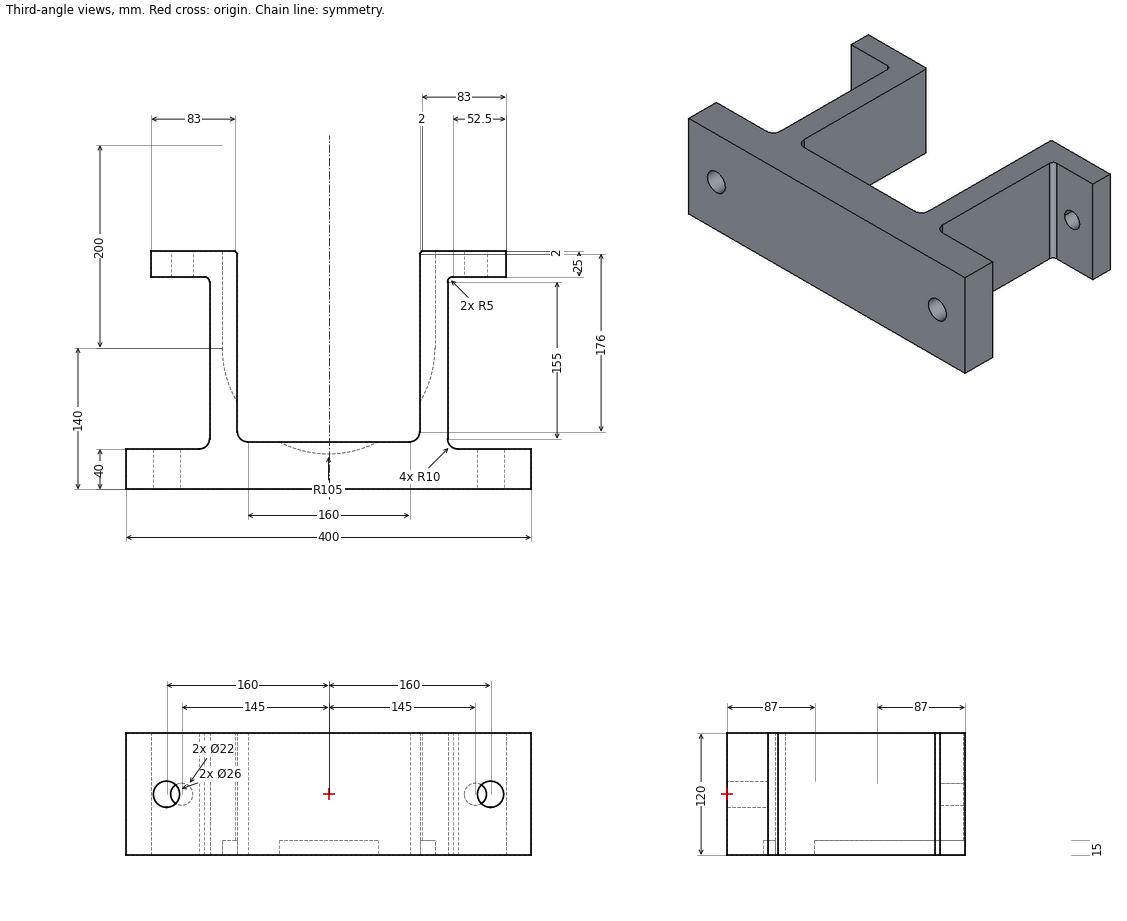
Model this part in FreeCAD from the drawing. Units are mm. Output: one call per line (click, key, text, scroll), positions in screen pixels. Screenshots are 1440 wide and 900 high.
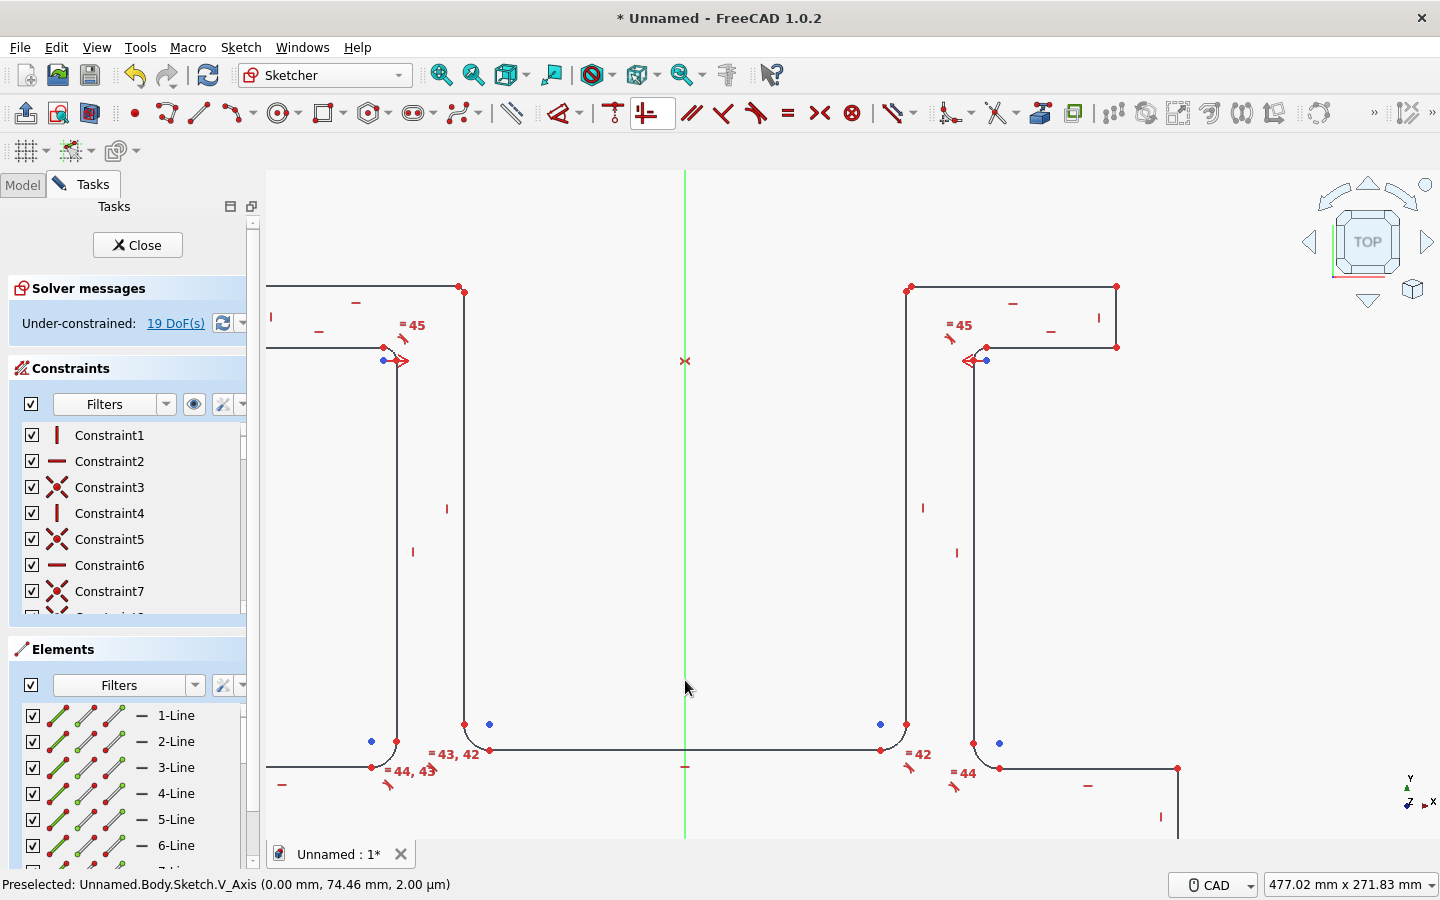
scroll(906, 291, up, 4)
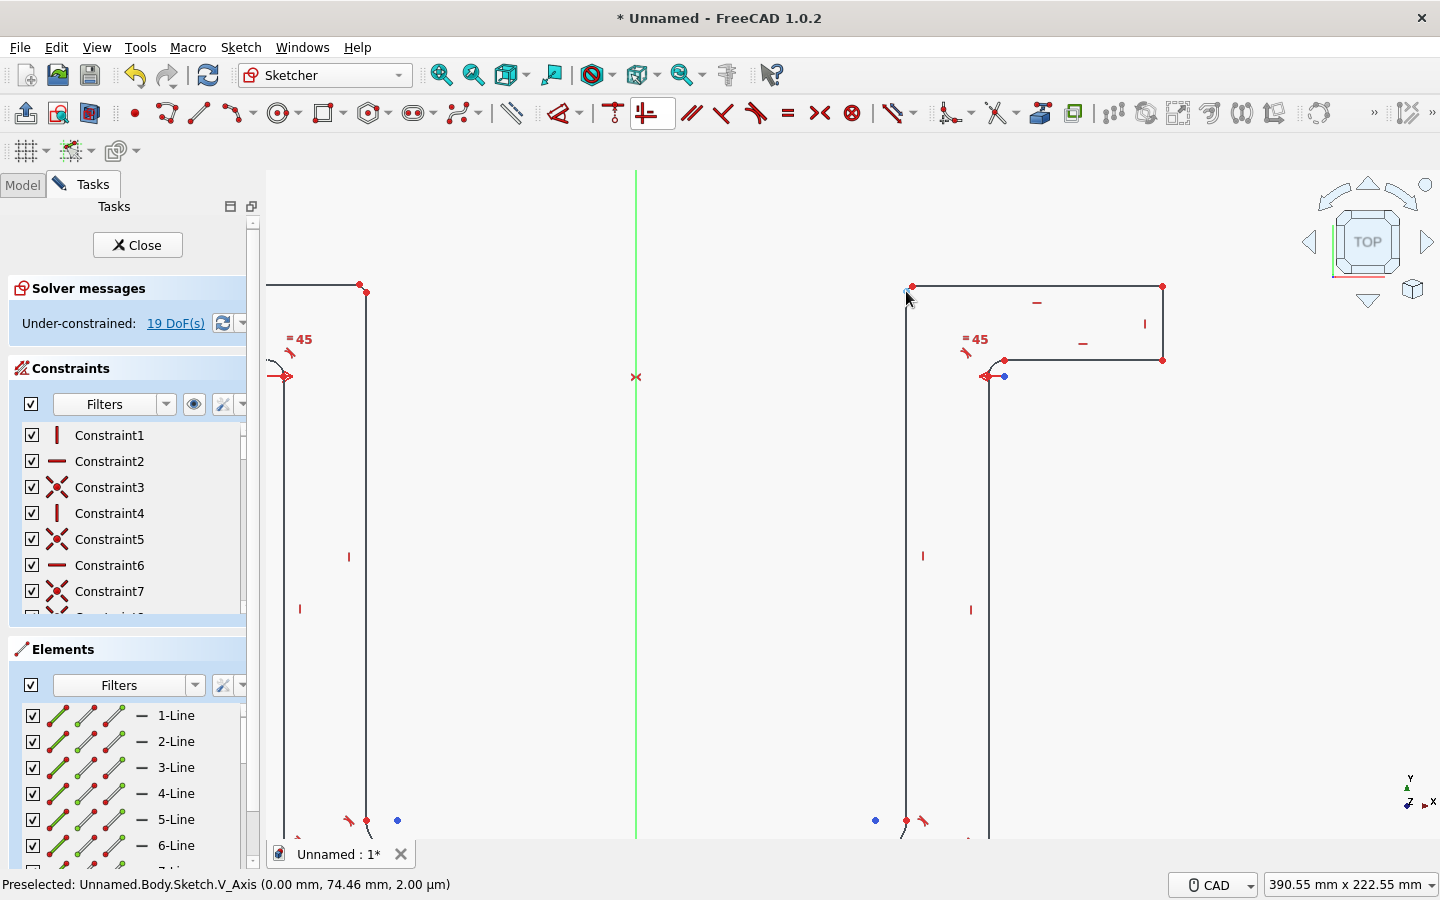
click(906, 291)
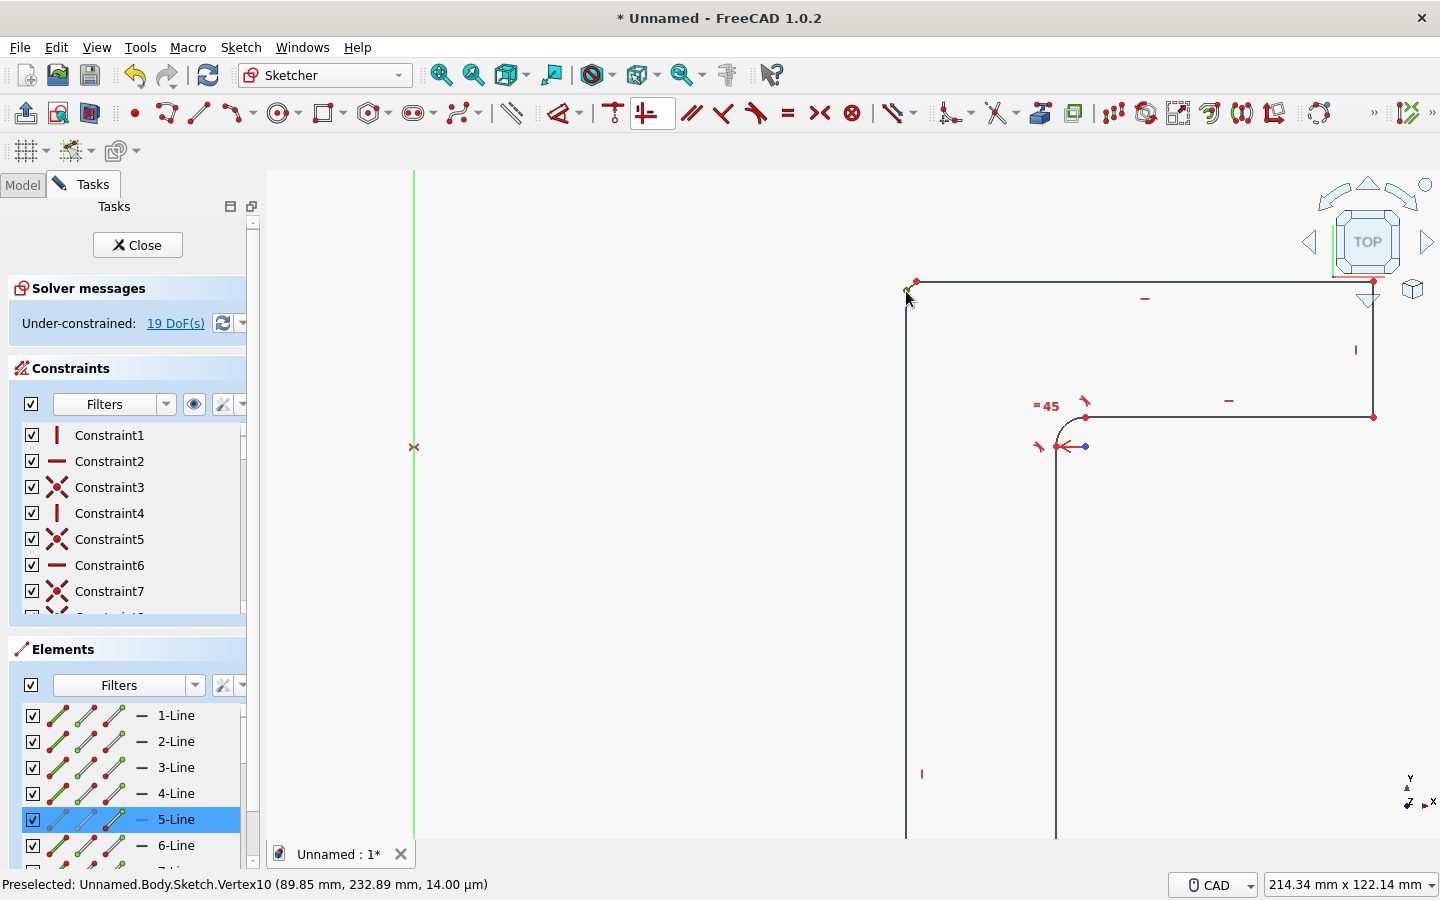
scroll(944, 324, down, 6)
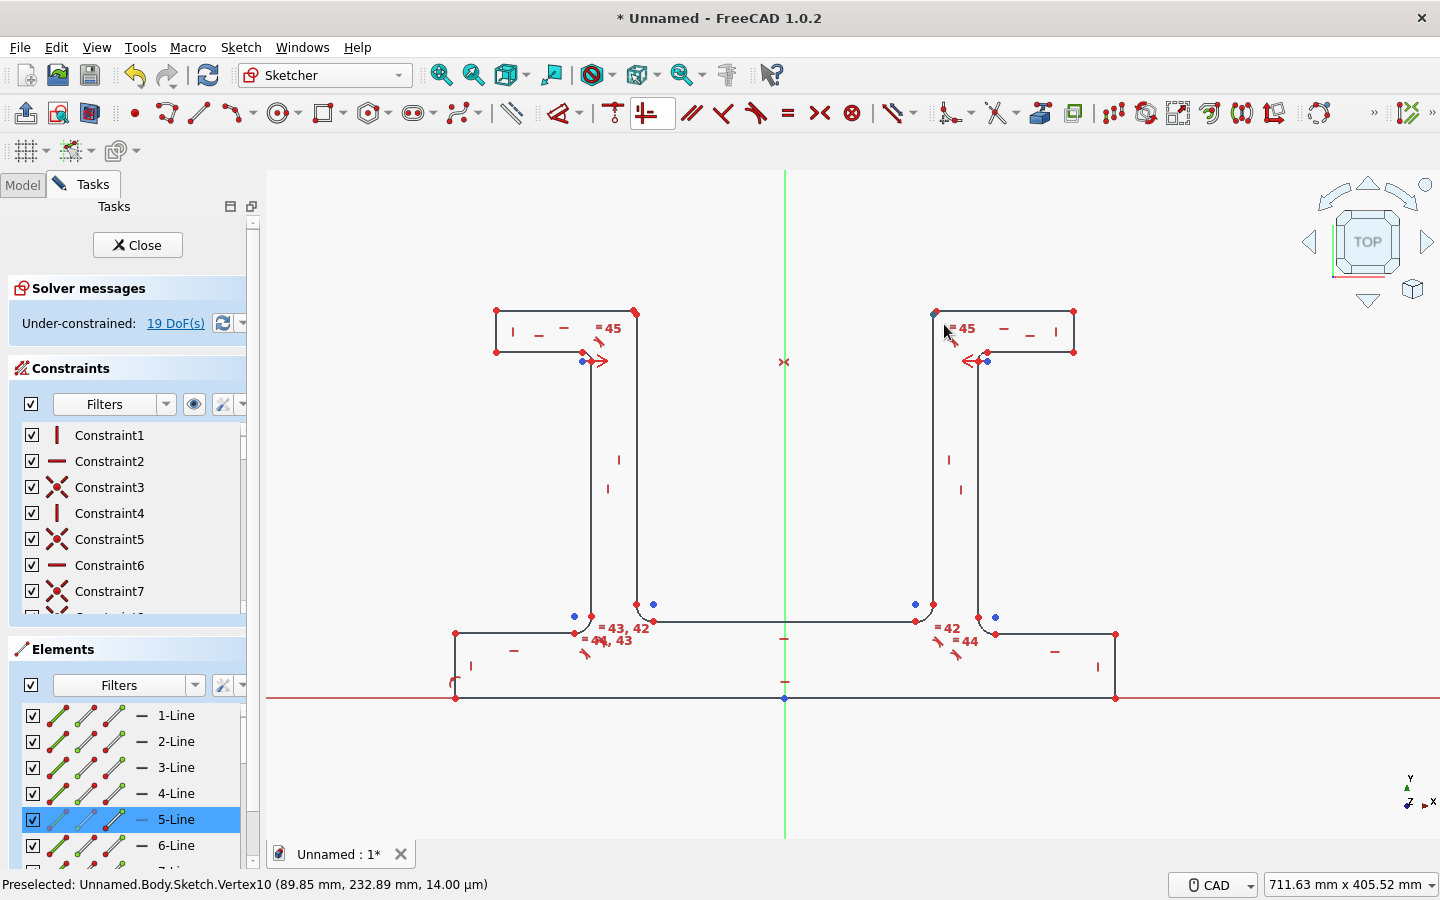
scroll(637, 315, up, 5)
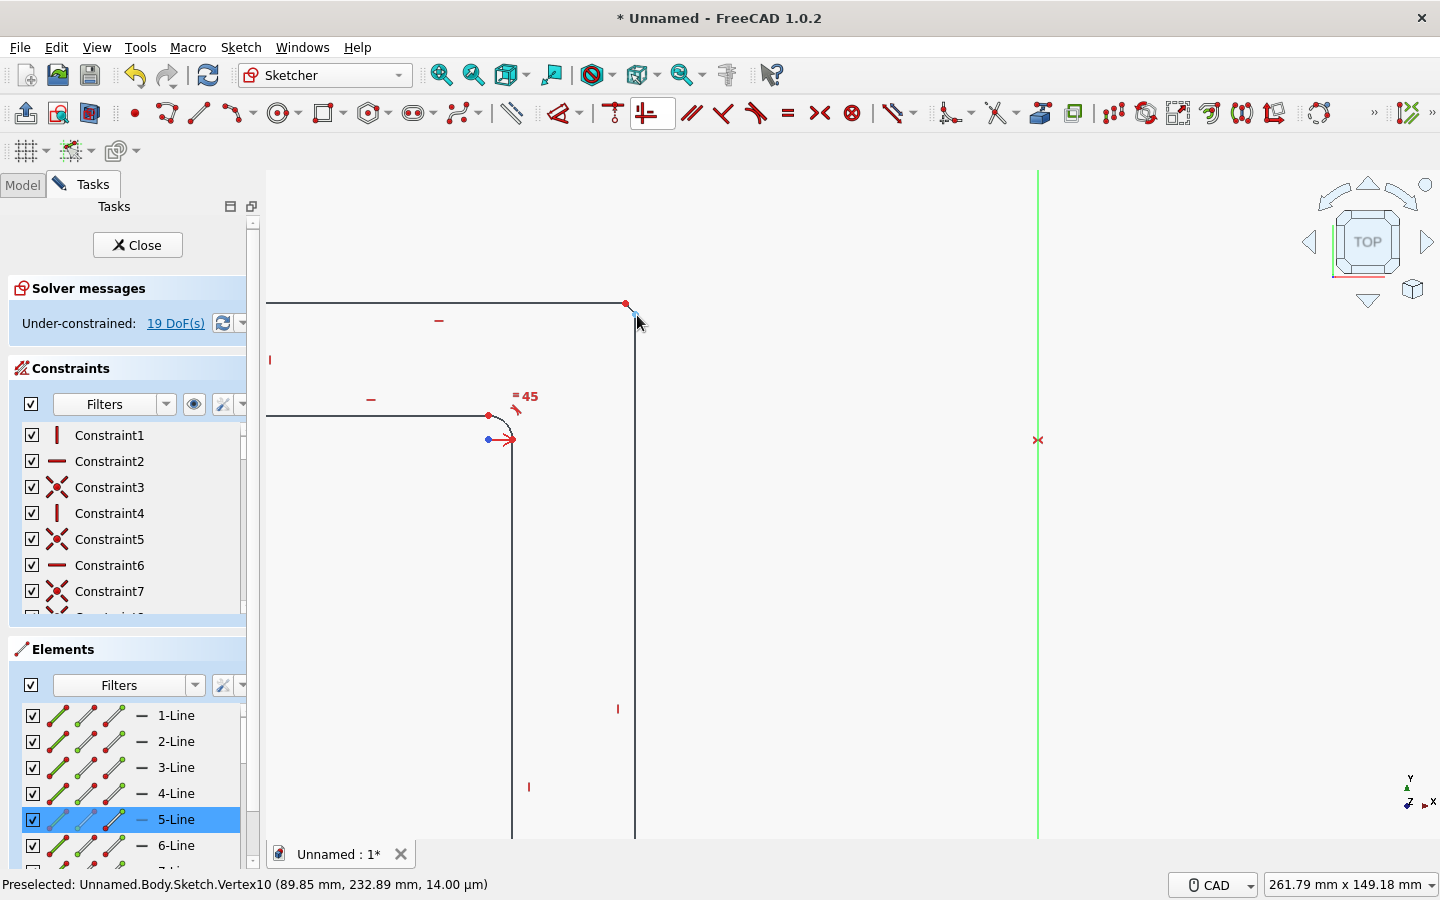
click(635, 315)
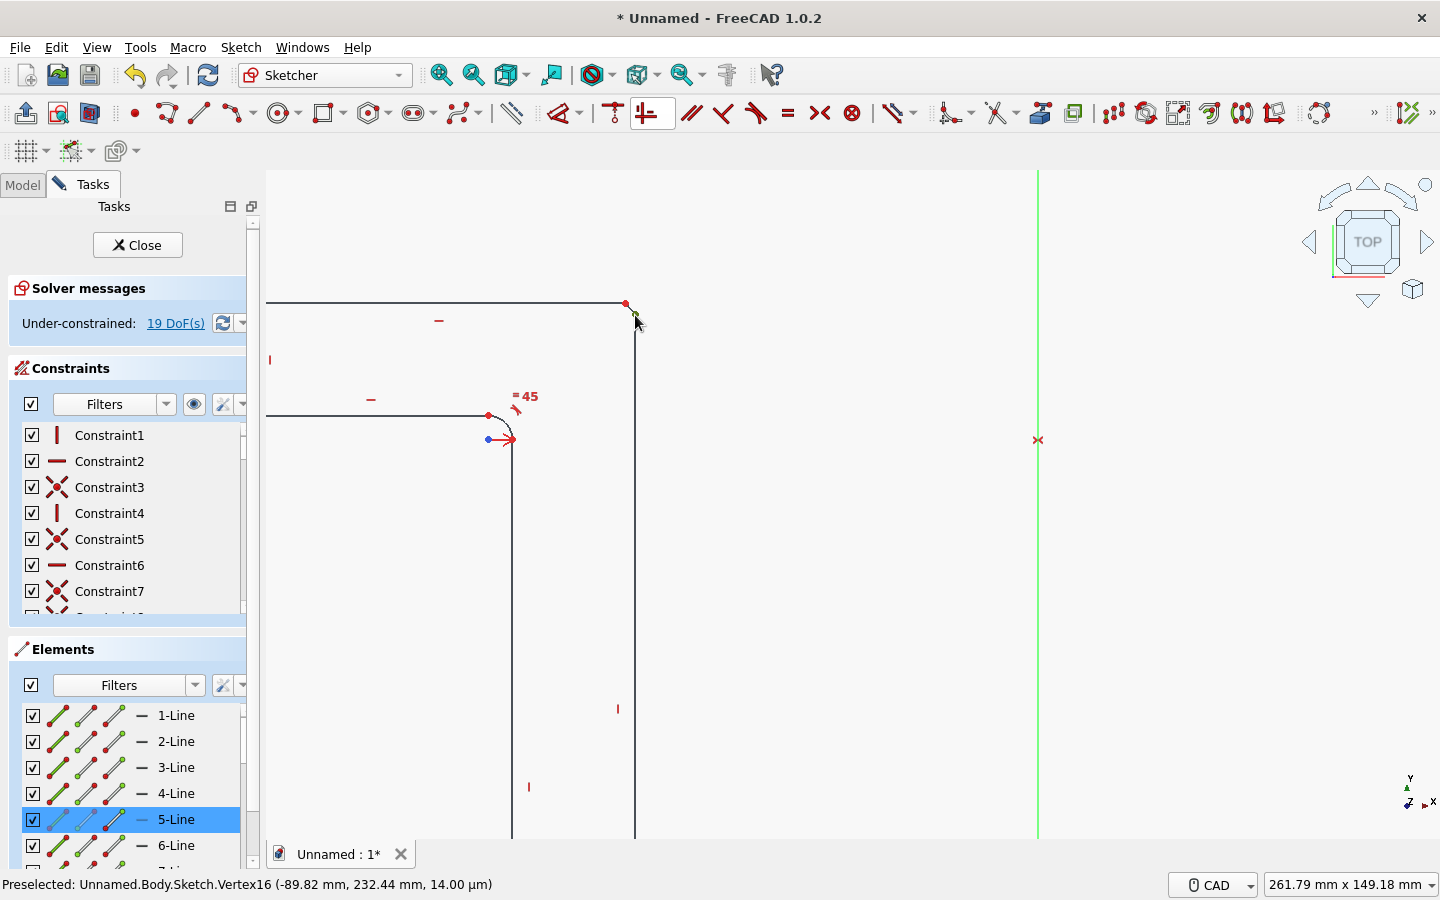
click(1038, 767)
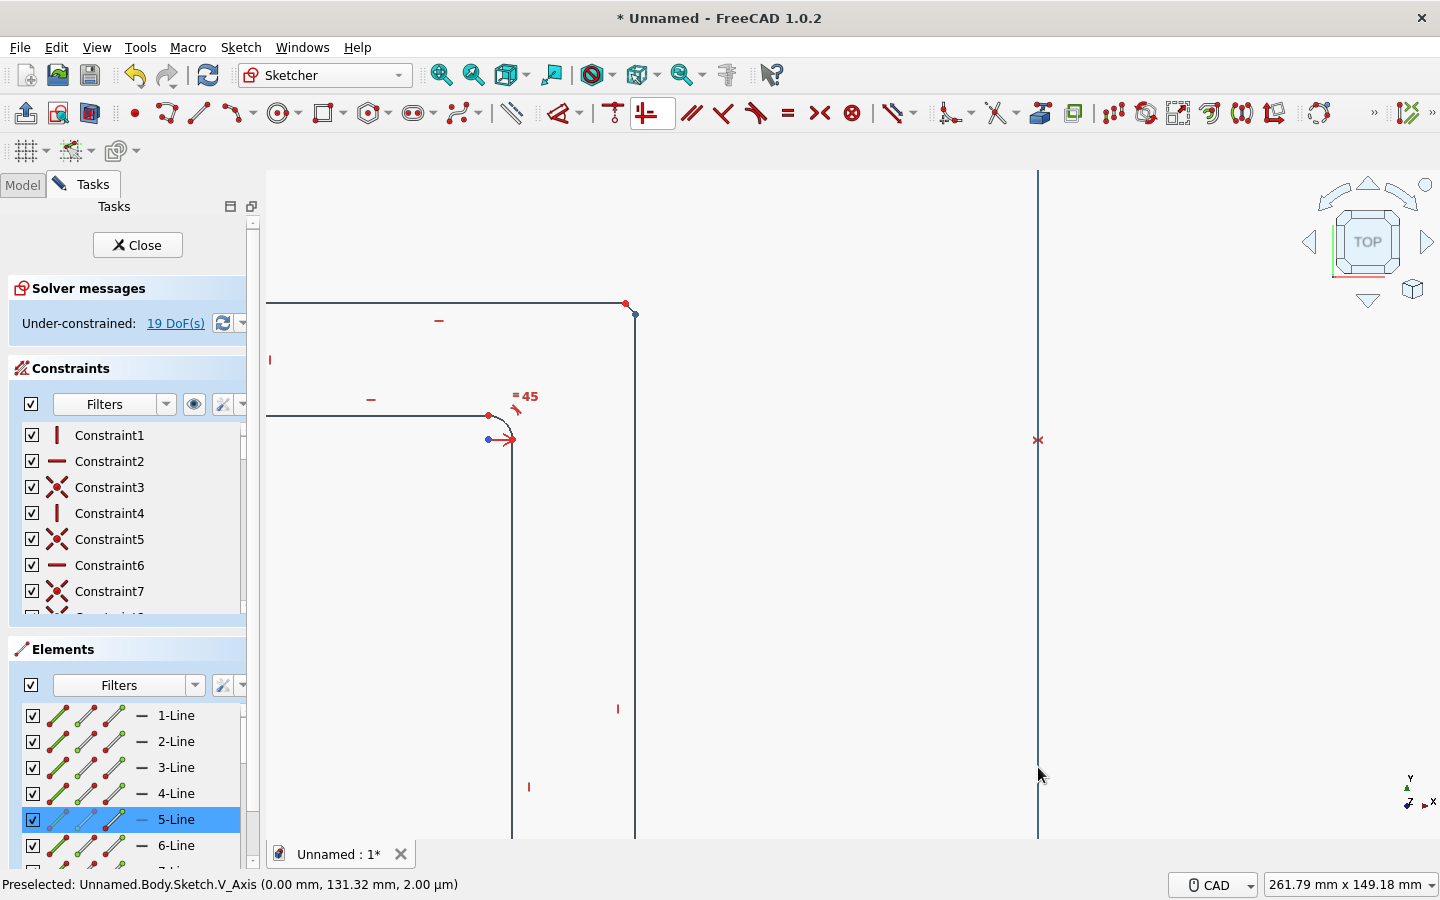
key(s)